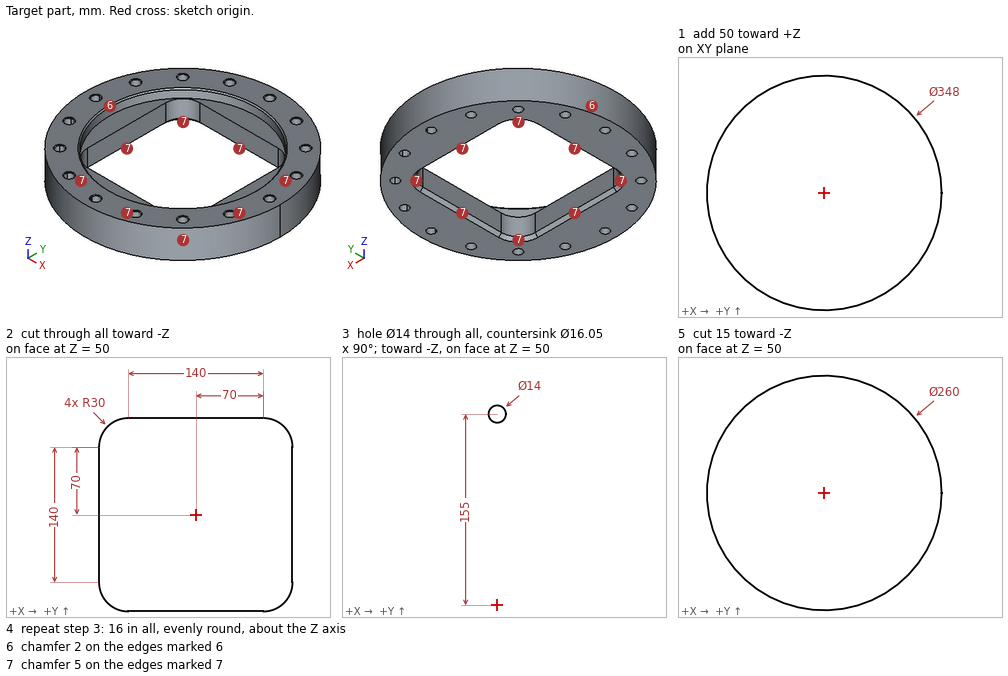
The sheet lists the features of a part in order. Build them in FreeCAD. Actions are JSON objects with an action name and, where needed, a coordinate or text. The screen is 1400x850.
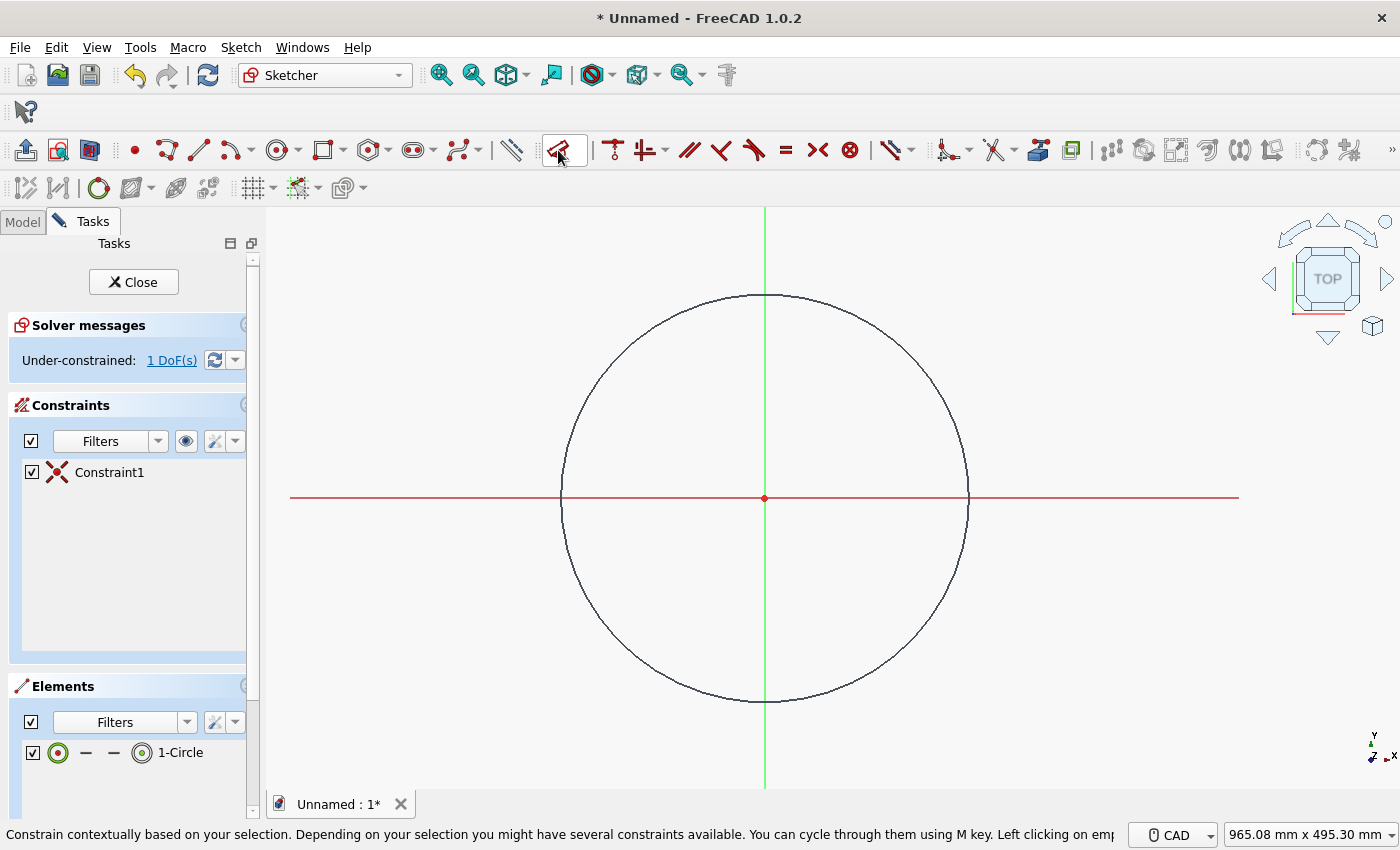
{"action": "left_click", "coordinate": [909, 354]}
{"action": "left_click", "coordinate": [932, 331]}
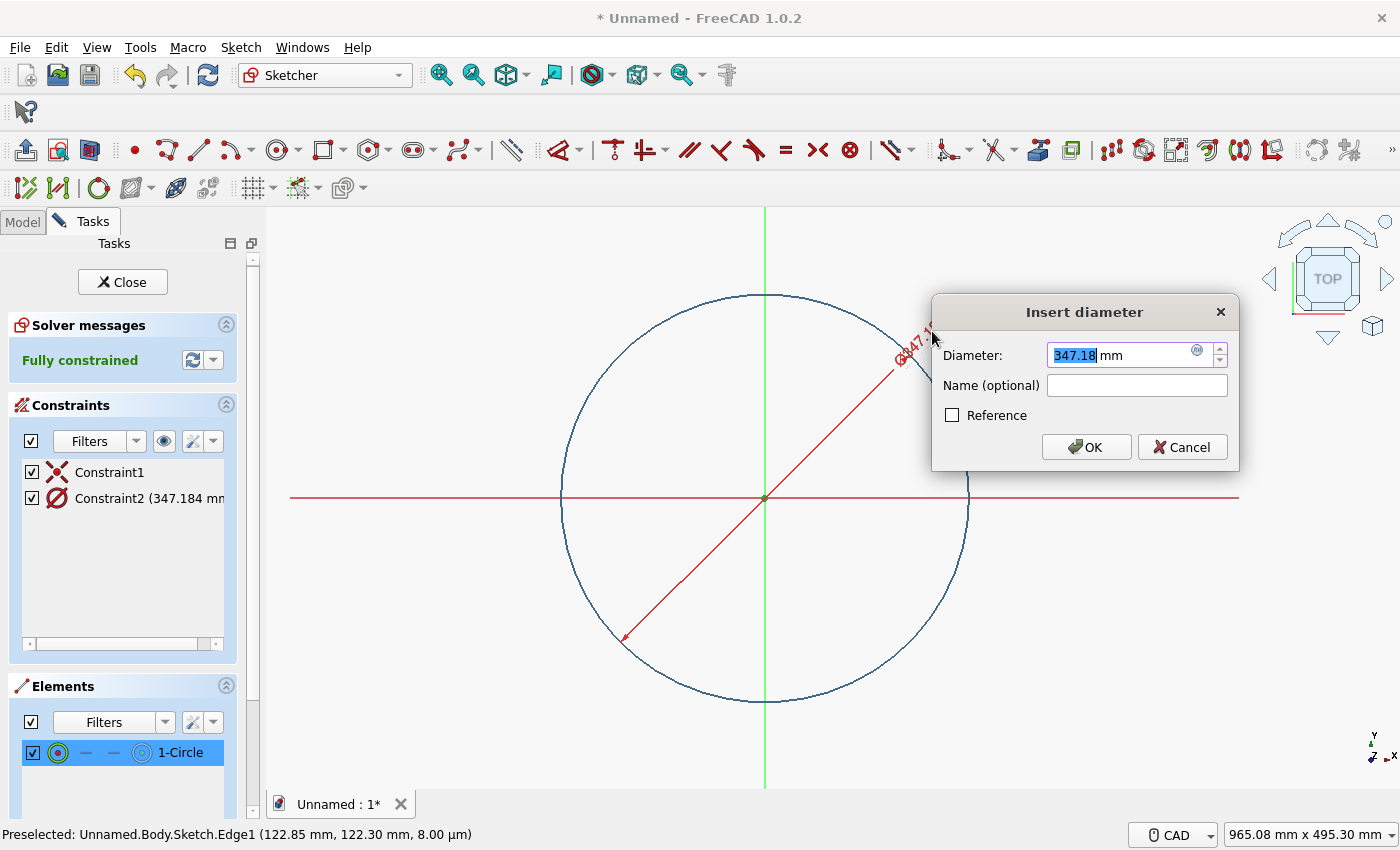
{"action": "type", "text": "348"}
{"action": "key", "text": "Return"}
{"action": "key", "text": "Escape"}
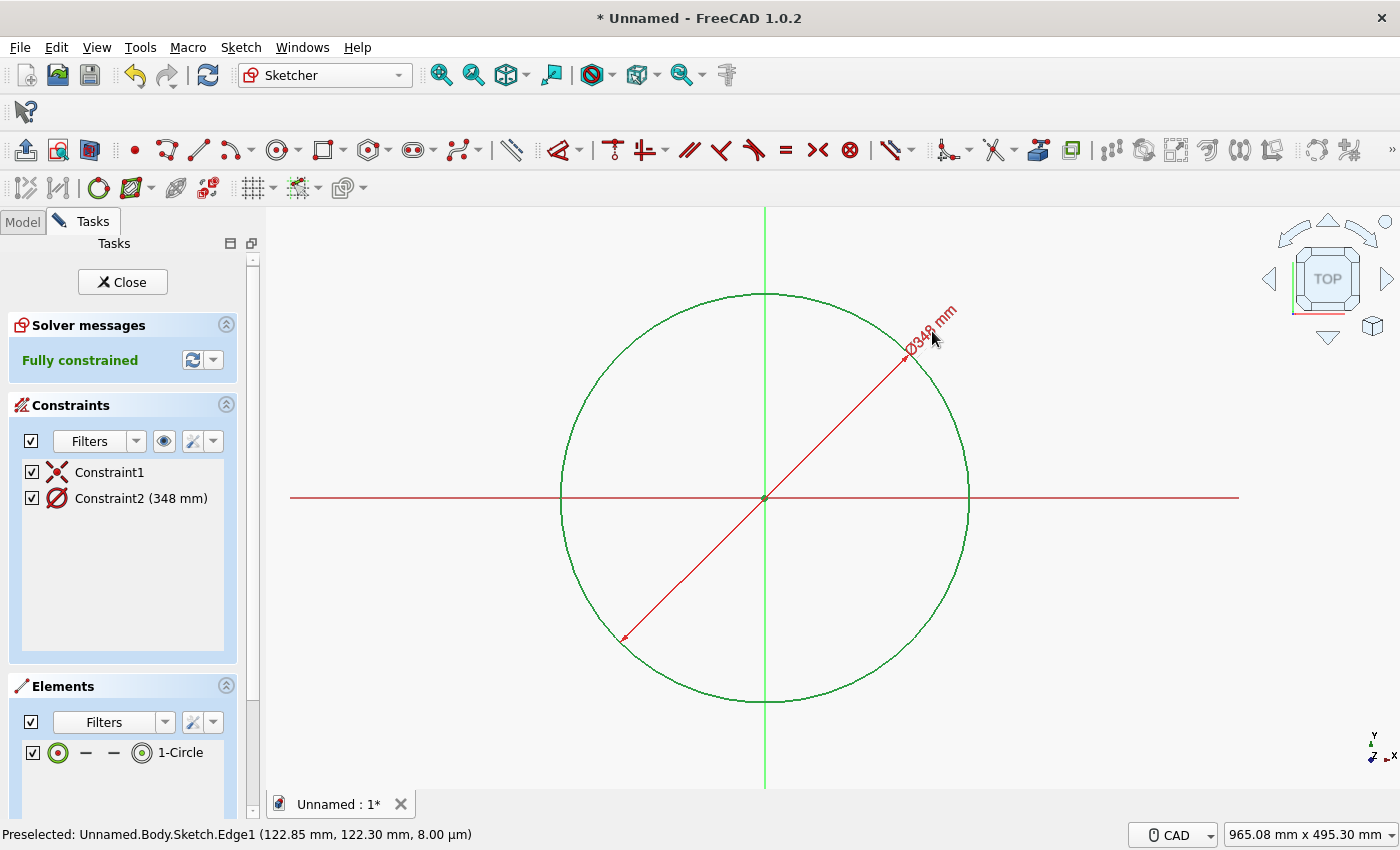
{"action": "left_click", "coordinate": [123, 282]}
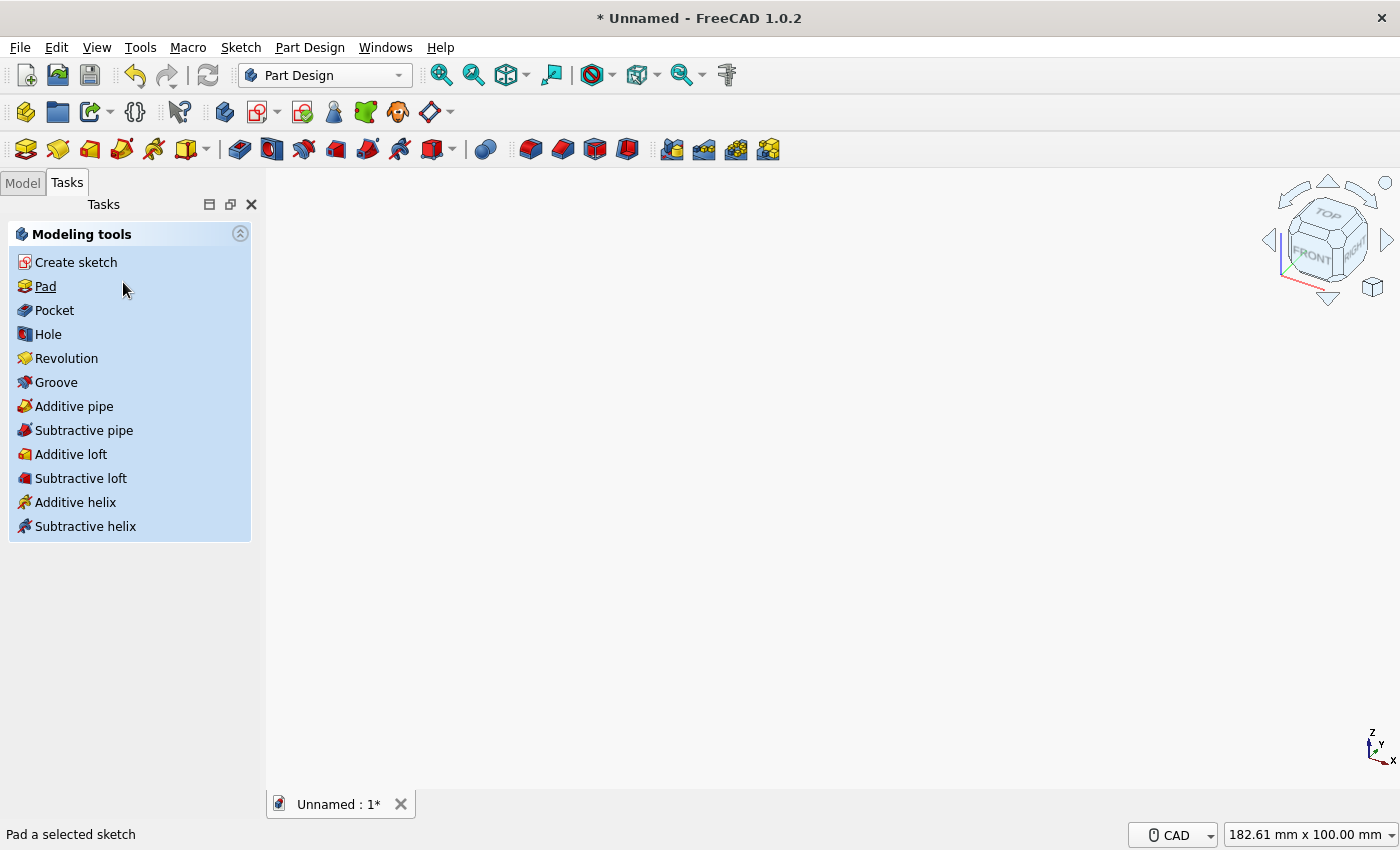
{"action": "left_click", "coordinate": [26, 150]}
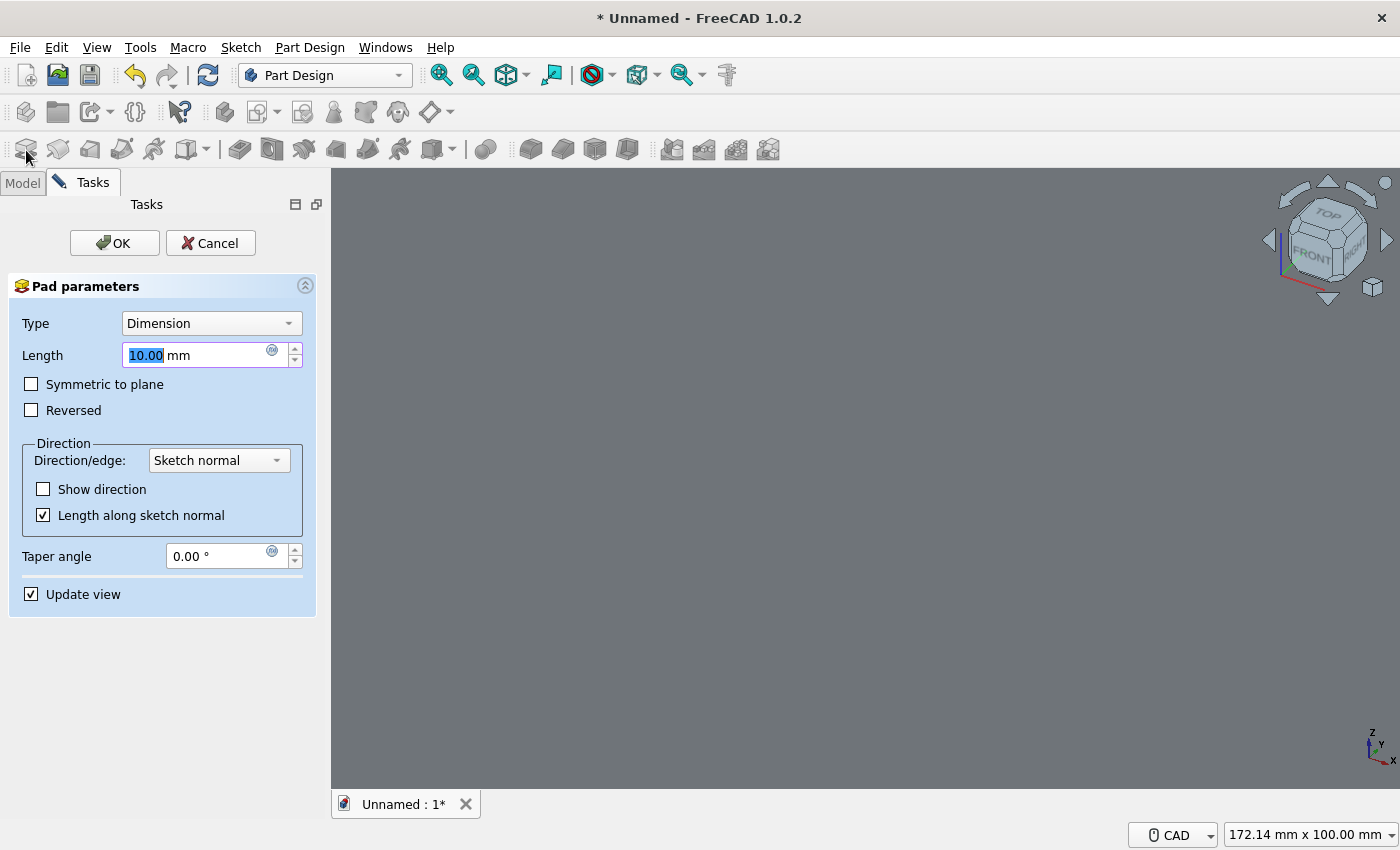
{"action": "type", "text": "50"}
{"action": "key", "text": "Tab"}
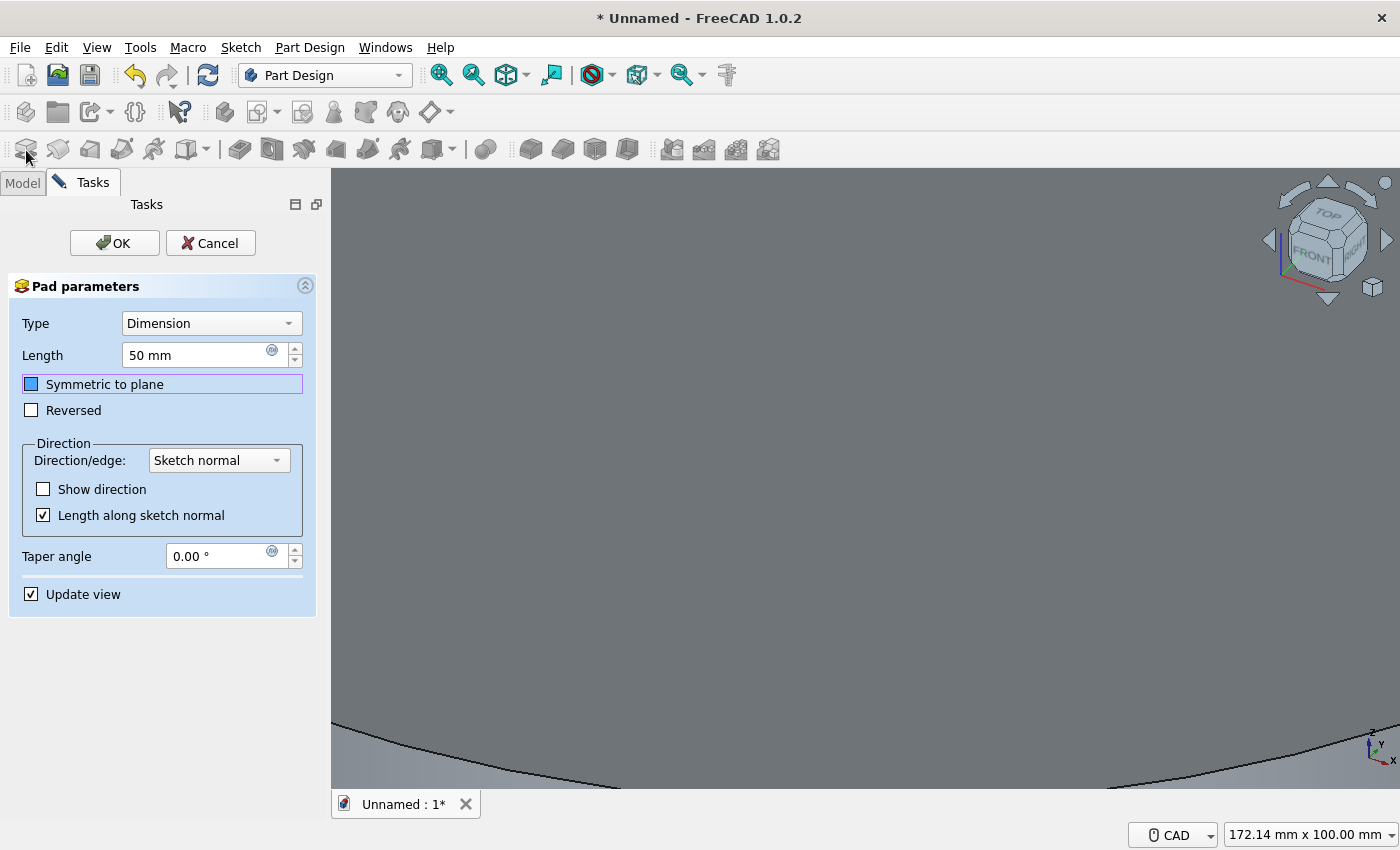
{"action": "left_click", "coordinate": [115, 243]}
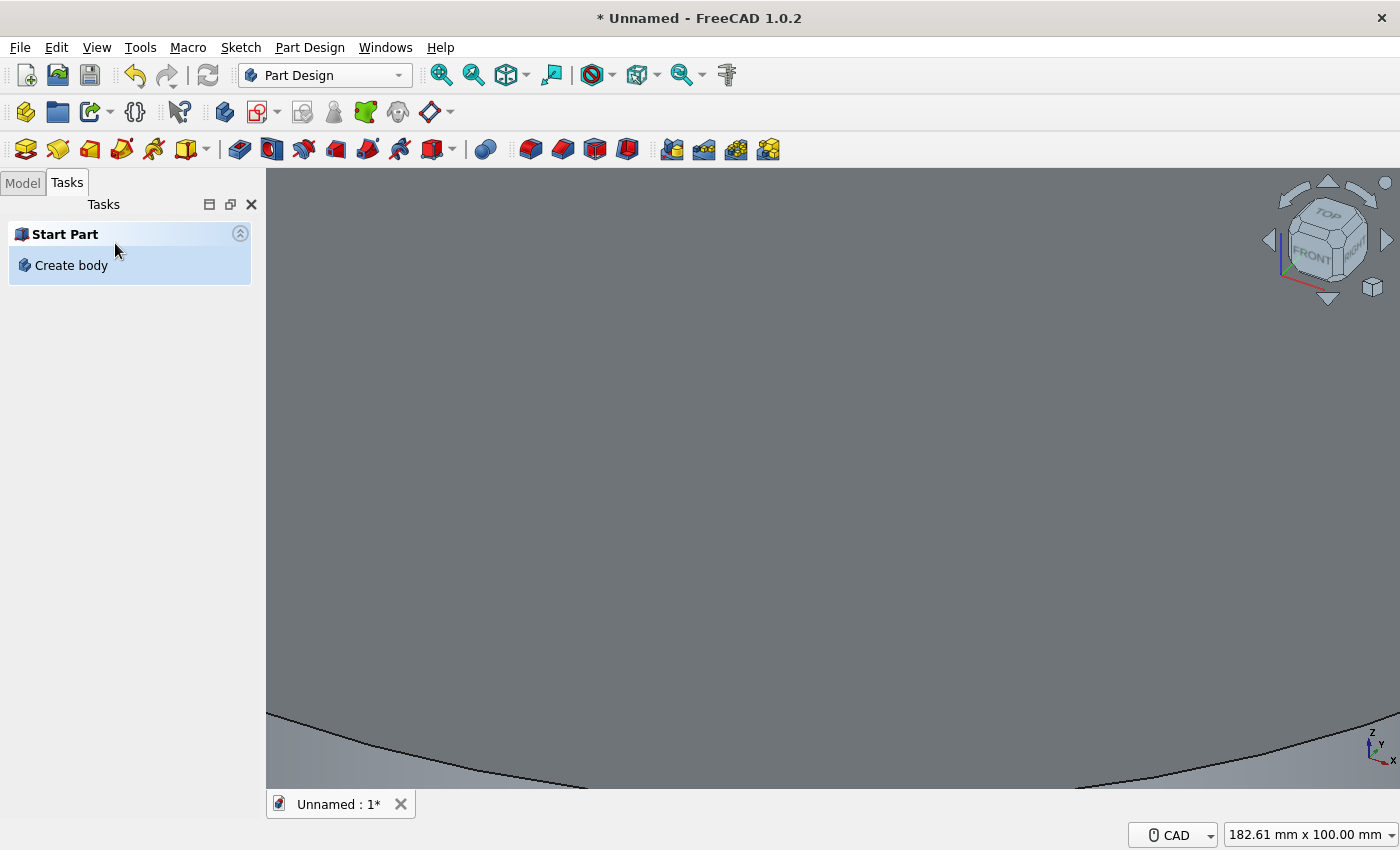
{"action": "left_click", "coordinate": [442, 76]}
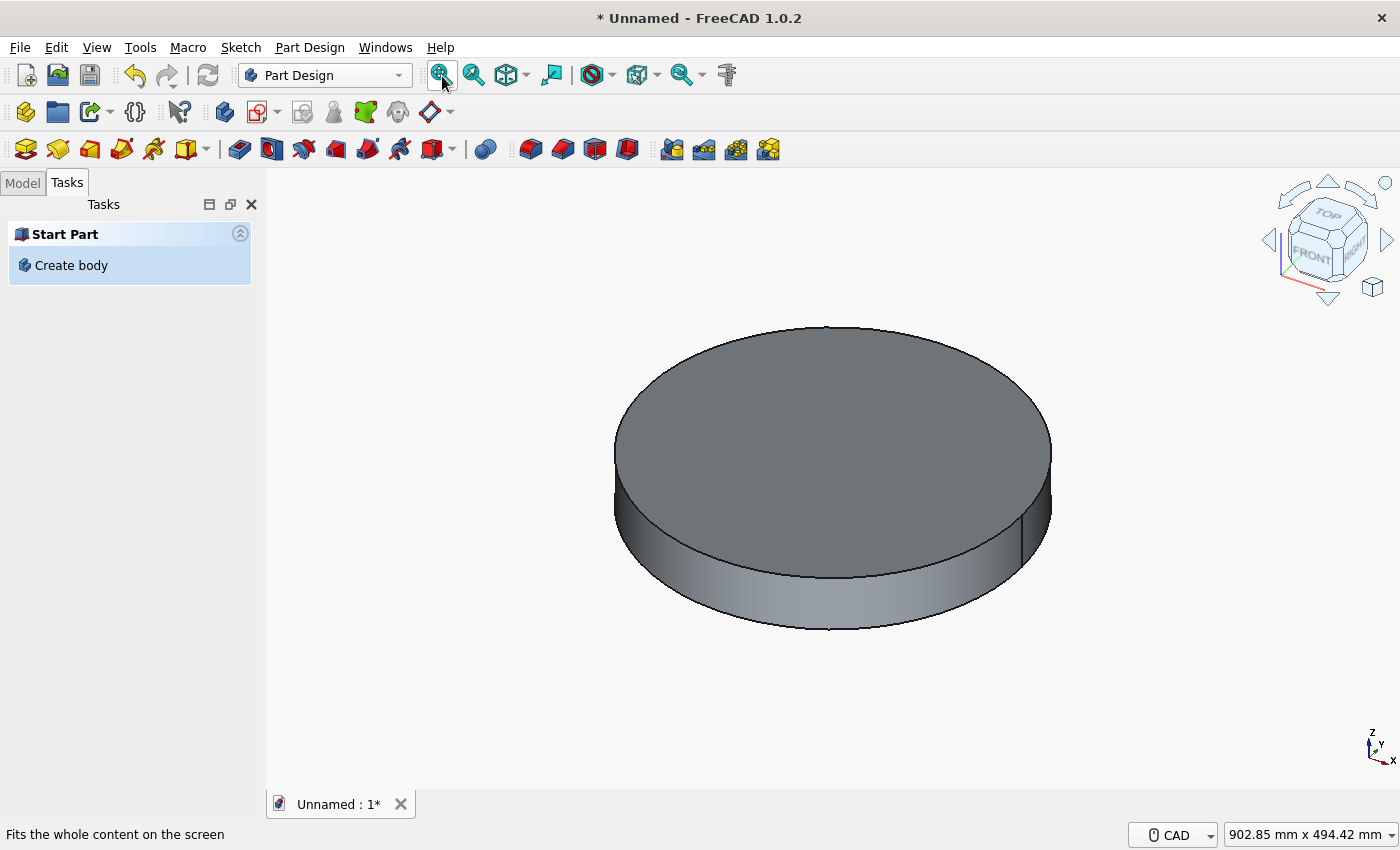
{"action": "left_click", "coordinate": [833, 452]}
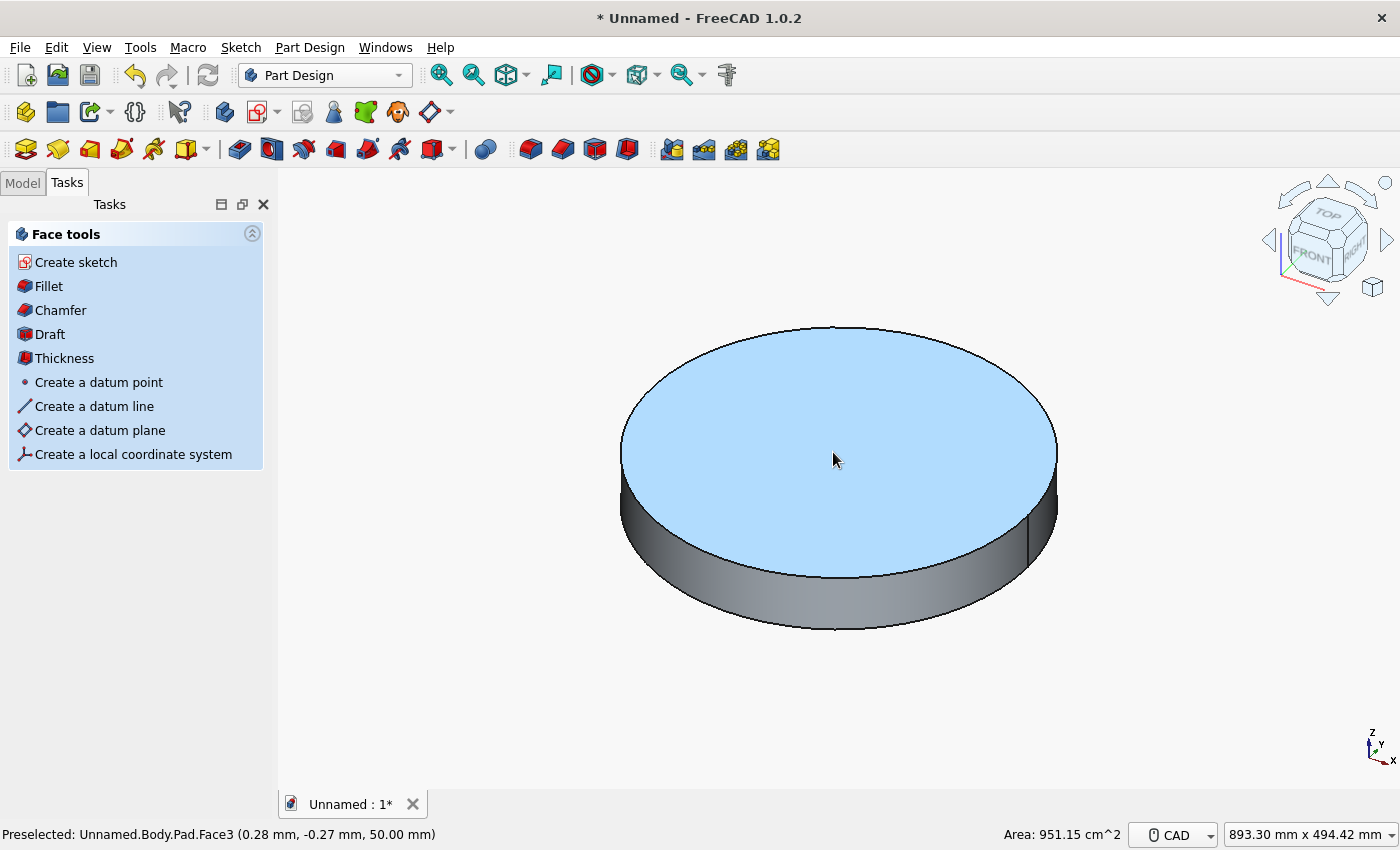
{"action": "left_click", "coordinate": [258, 112]}